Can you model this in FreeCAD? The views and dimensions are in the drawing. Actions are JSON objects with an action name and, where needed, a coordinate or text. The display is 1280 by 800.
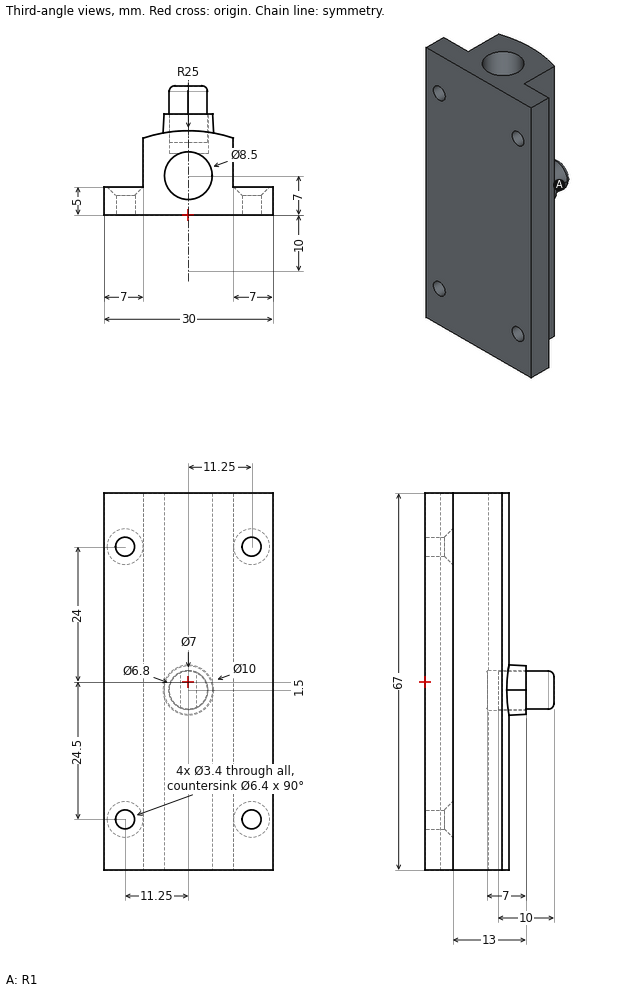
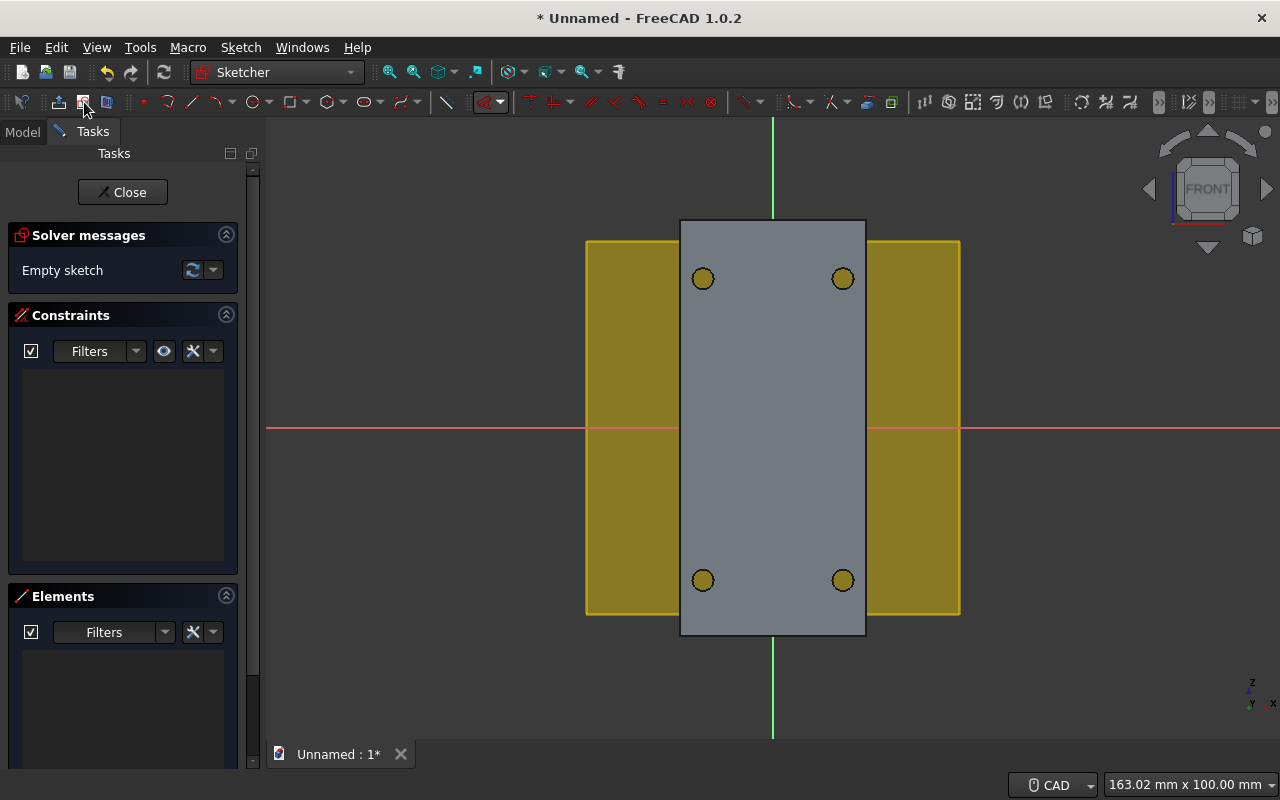
{"action": "scroll", "coordinate": [782, 438], "scroll_direction": "up", "scroll_amount": 11}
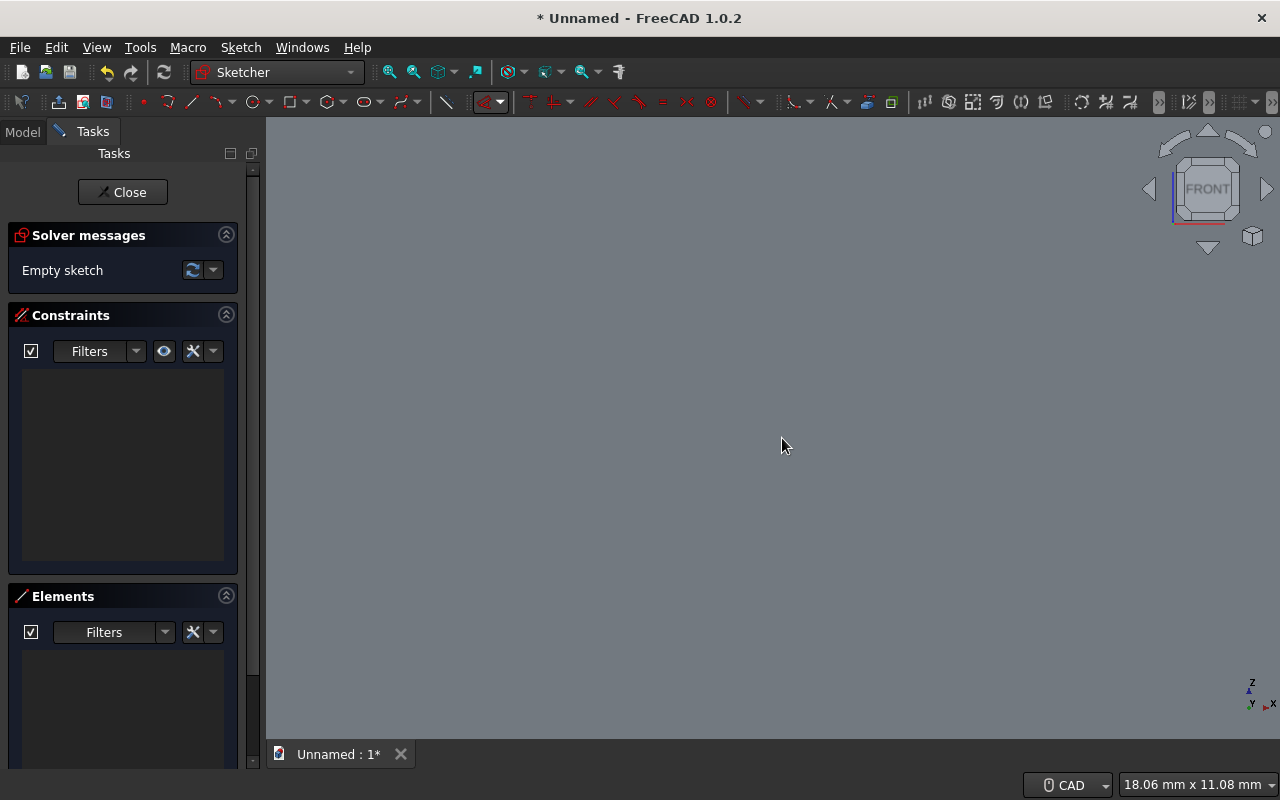
{"action": "key", "text": "g c"}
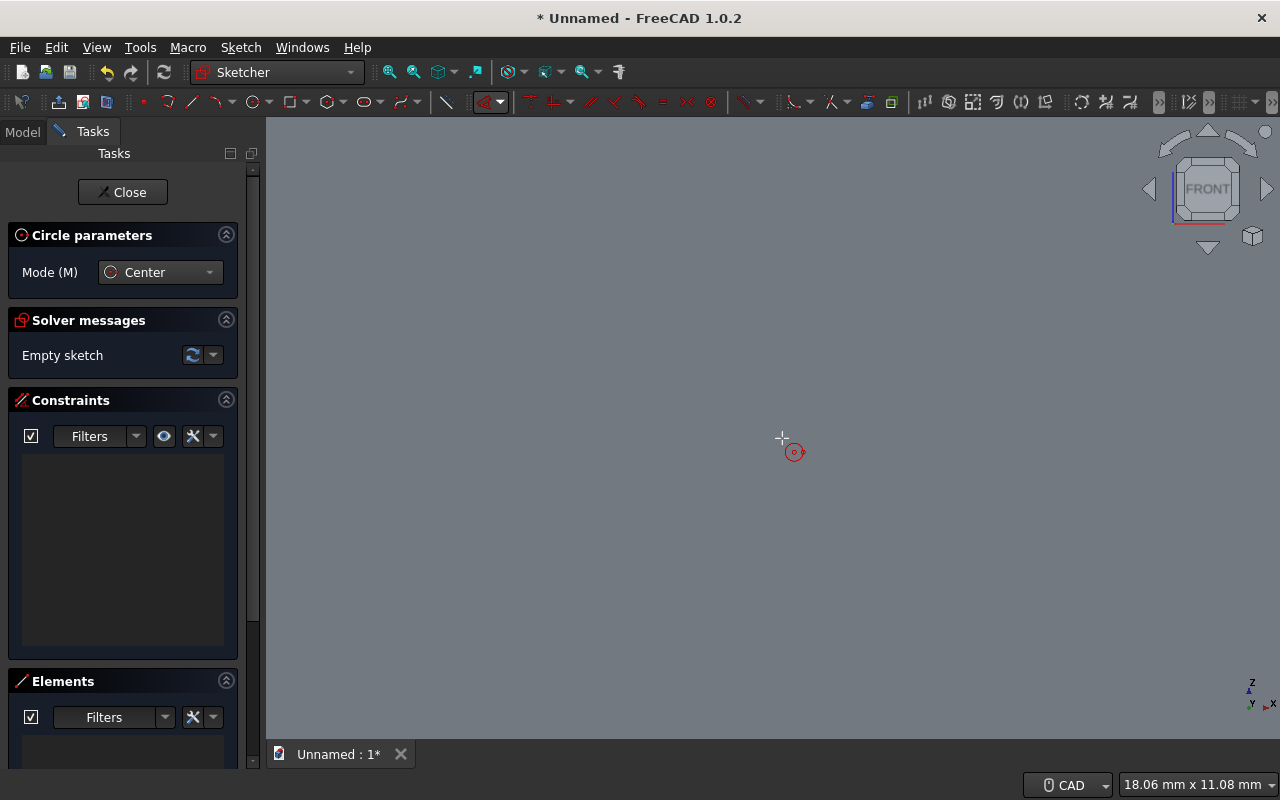
{"action": "left_click", "coordinate": [697, 428]}
{"action": "left_click", "coordinate": [832, 293]}
{"action": "key", "text": "Escape"}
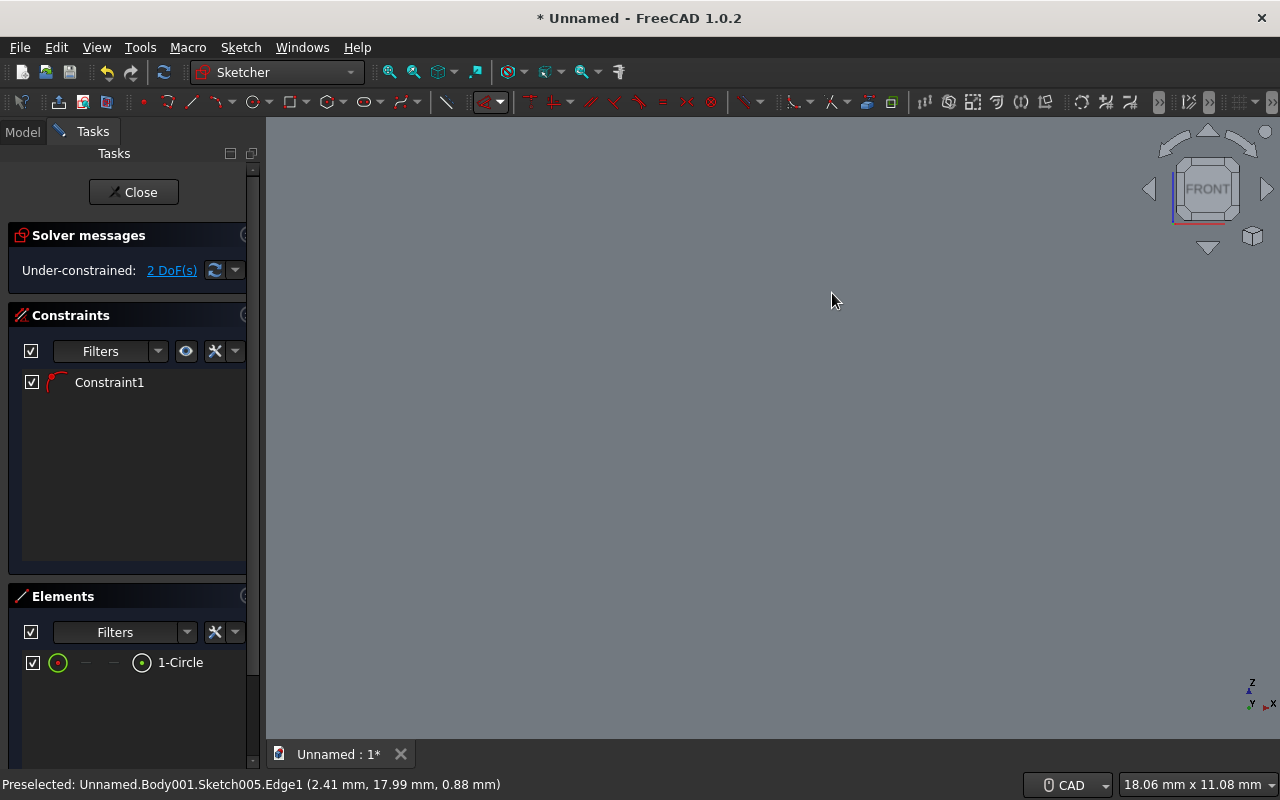
{"action": "left_click", "coordinate": [831, 293]}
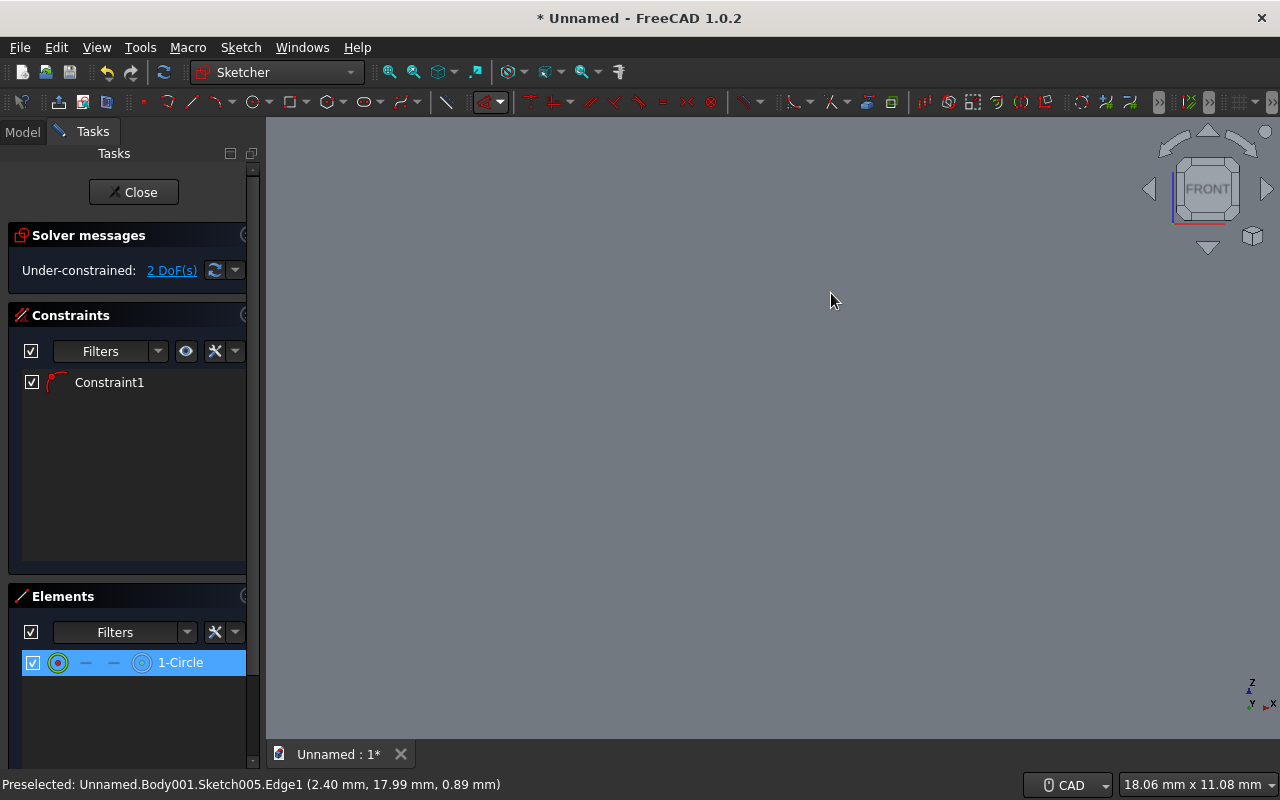
{"action": "left_click", "coordinate": [502, 102]}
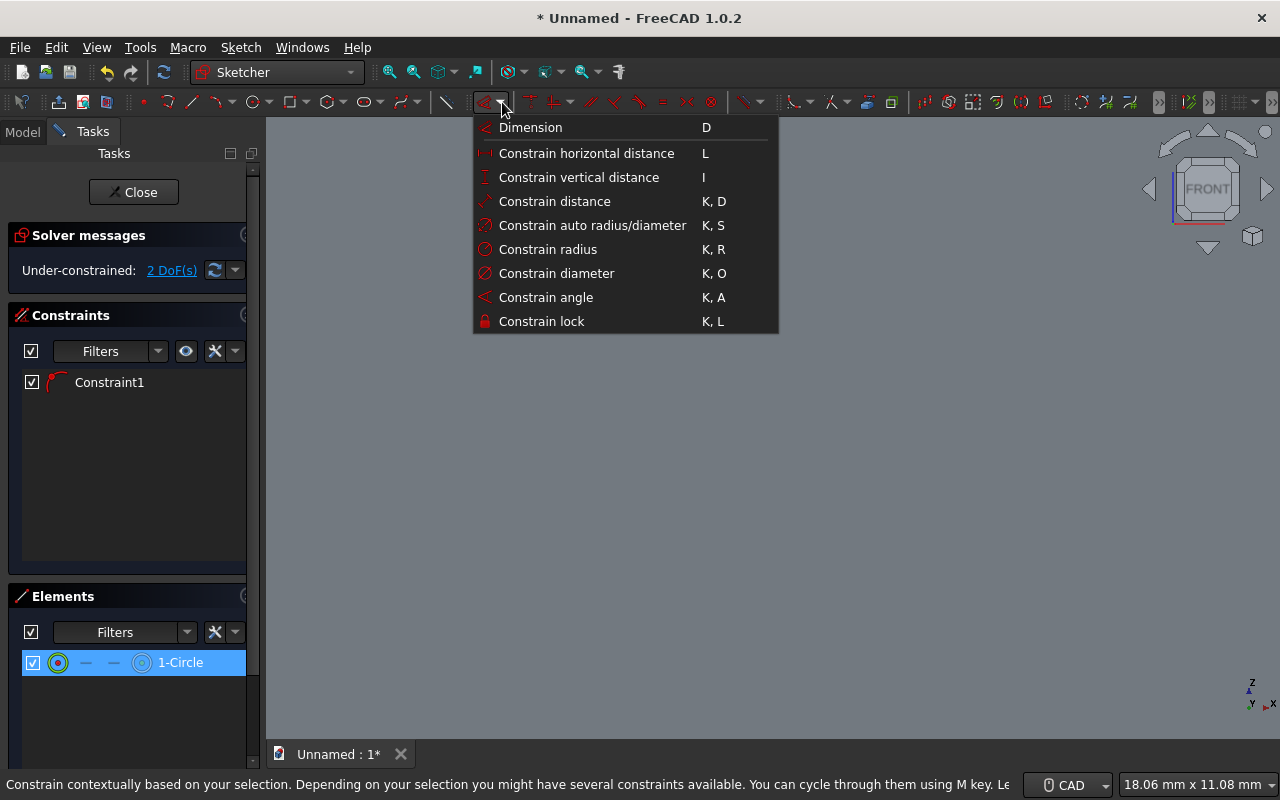
{"action": "left_click", "coordinate": [626, 273]}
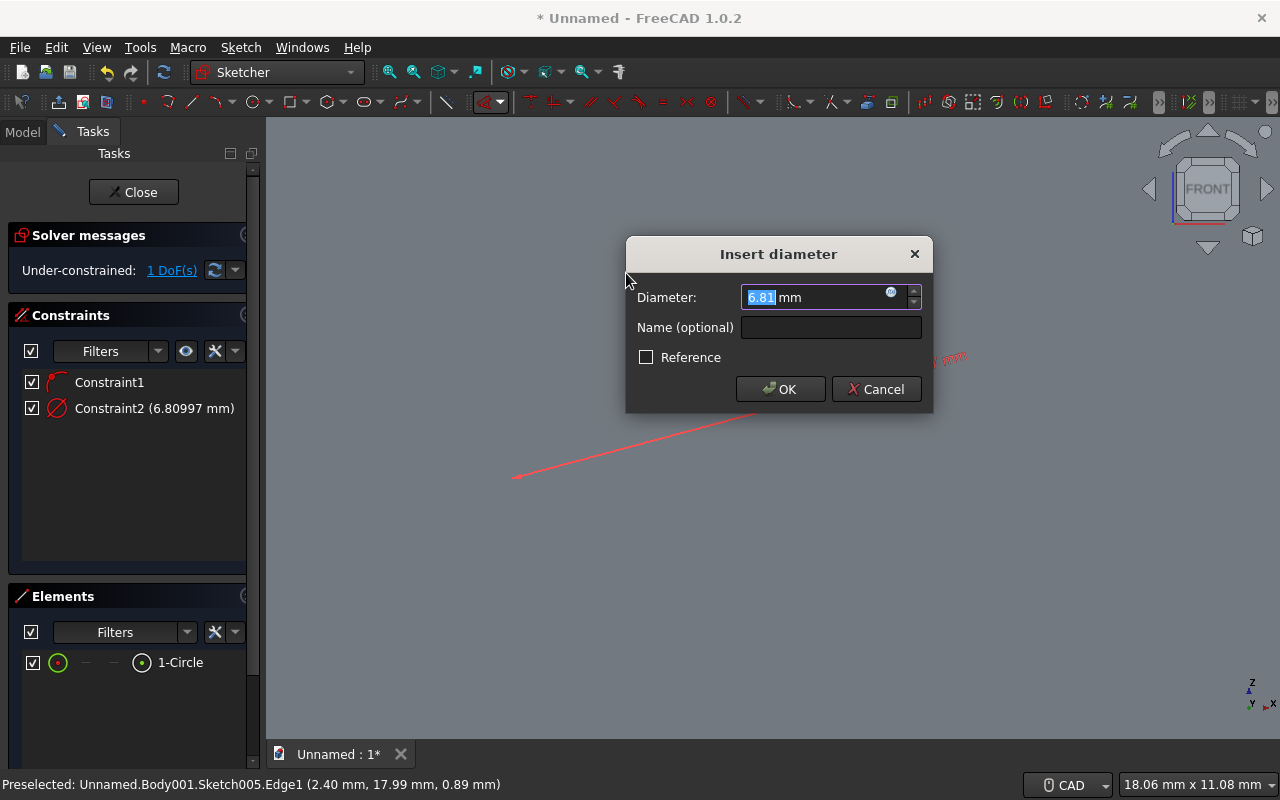
{"action": "type", "text": "6.8"}
{"action": "key", "text": "Return"}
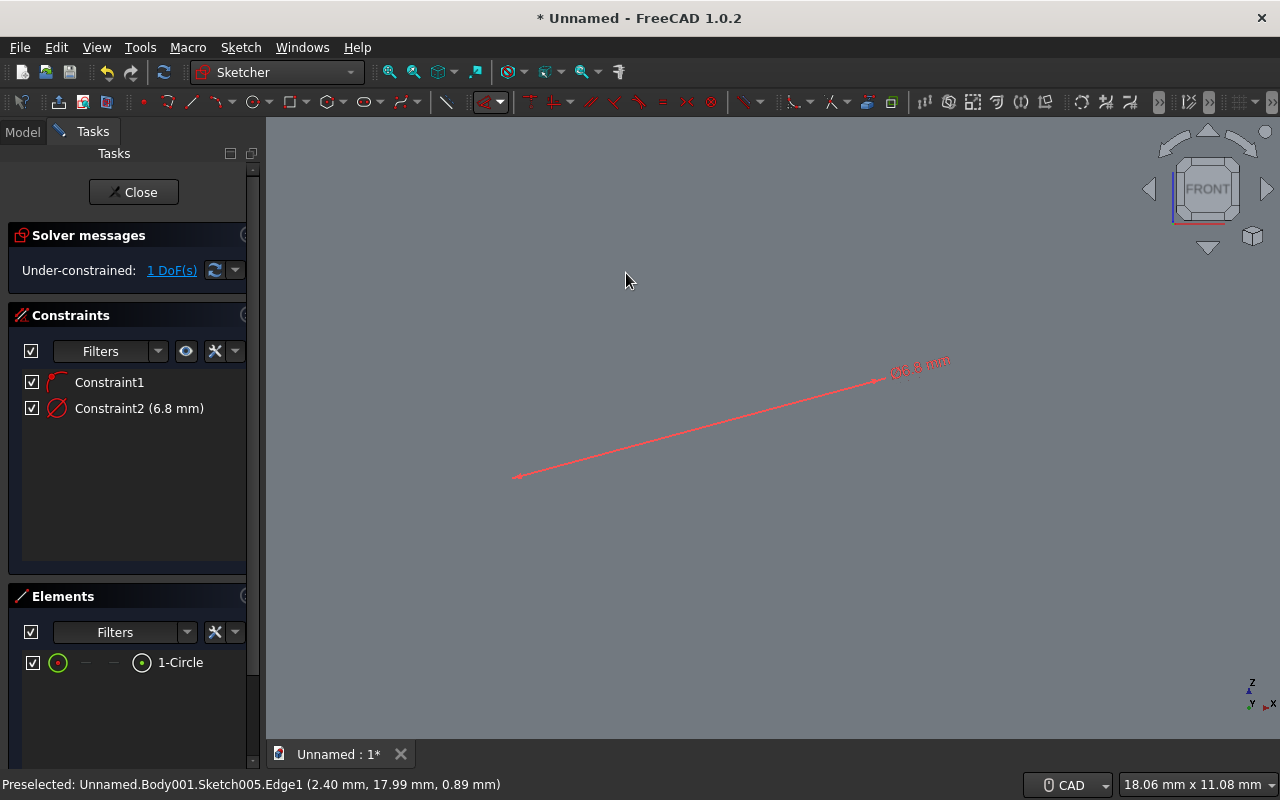
{"action": "left_click", "coordinate": [697, 429]}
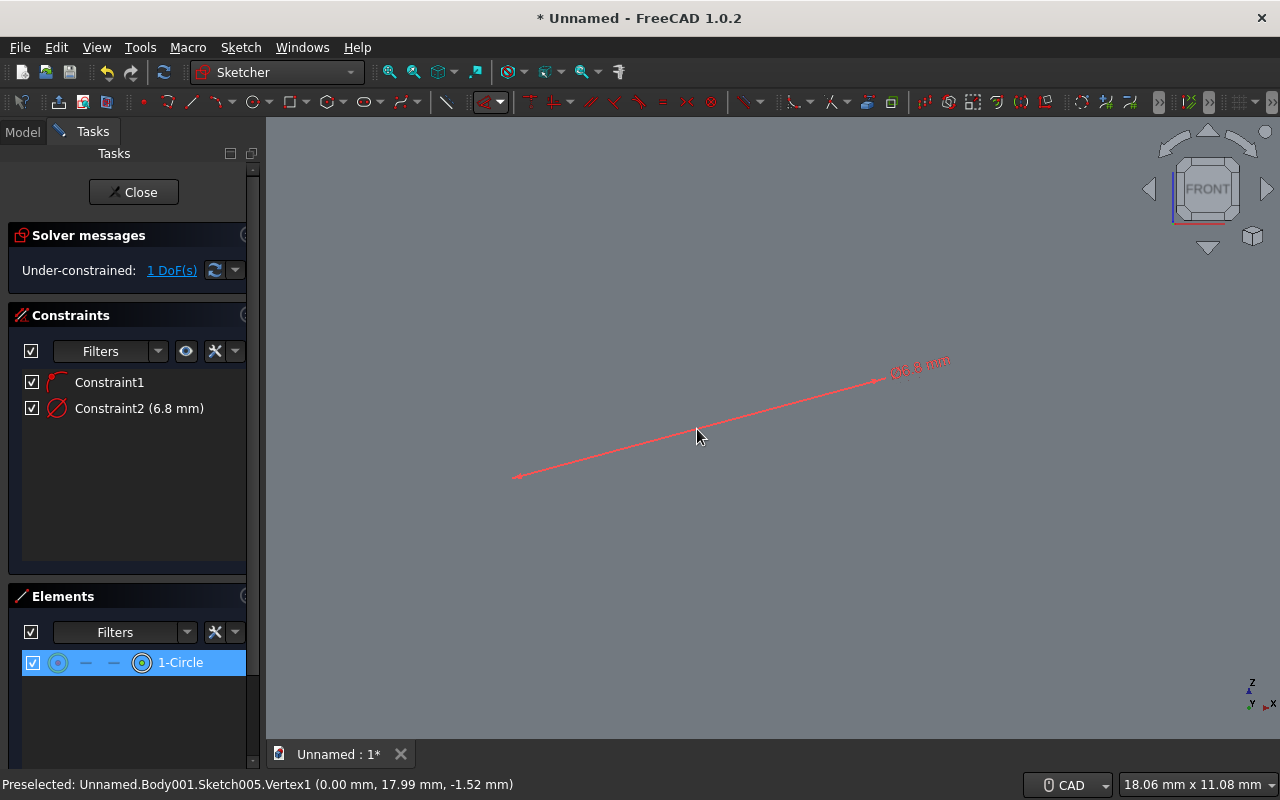
{"action": "left_click", "coordinate": [502, 102]}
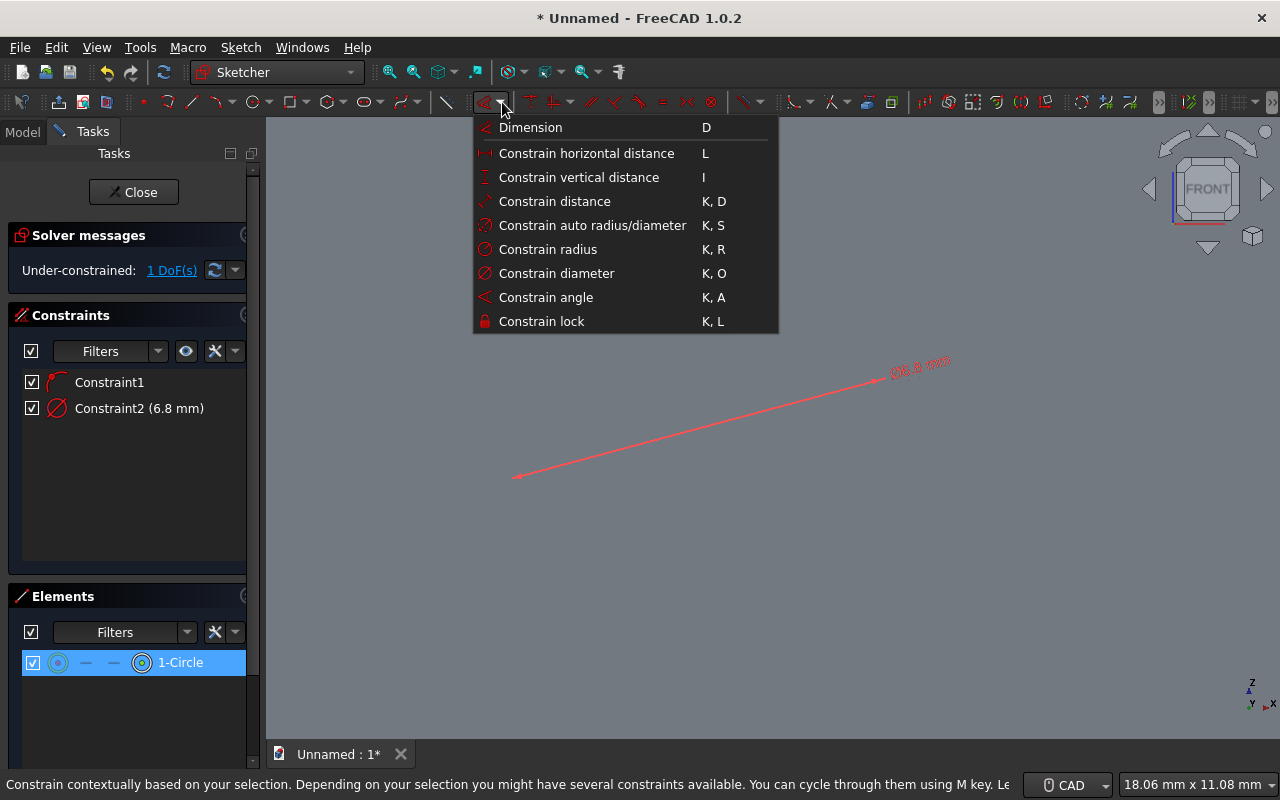
{"action": "left_click", "coordinate": [626, 177]}